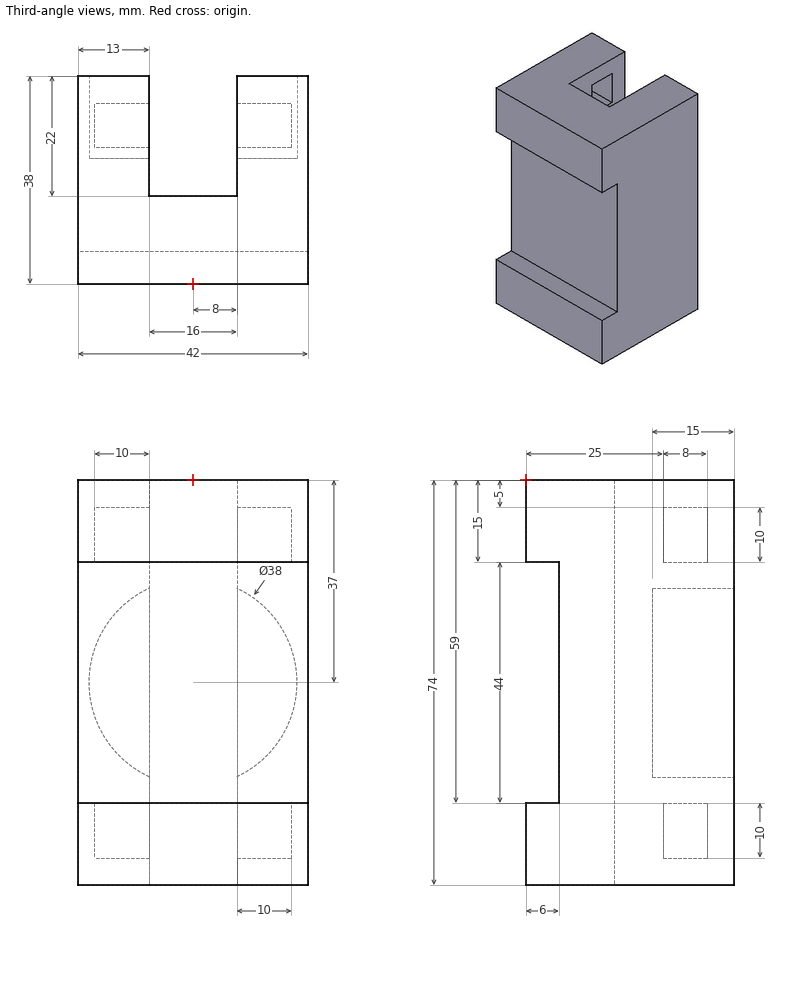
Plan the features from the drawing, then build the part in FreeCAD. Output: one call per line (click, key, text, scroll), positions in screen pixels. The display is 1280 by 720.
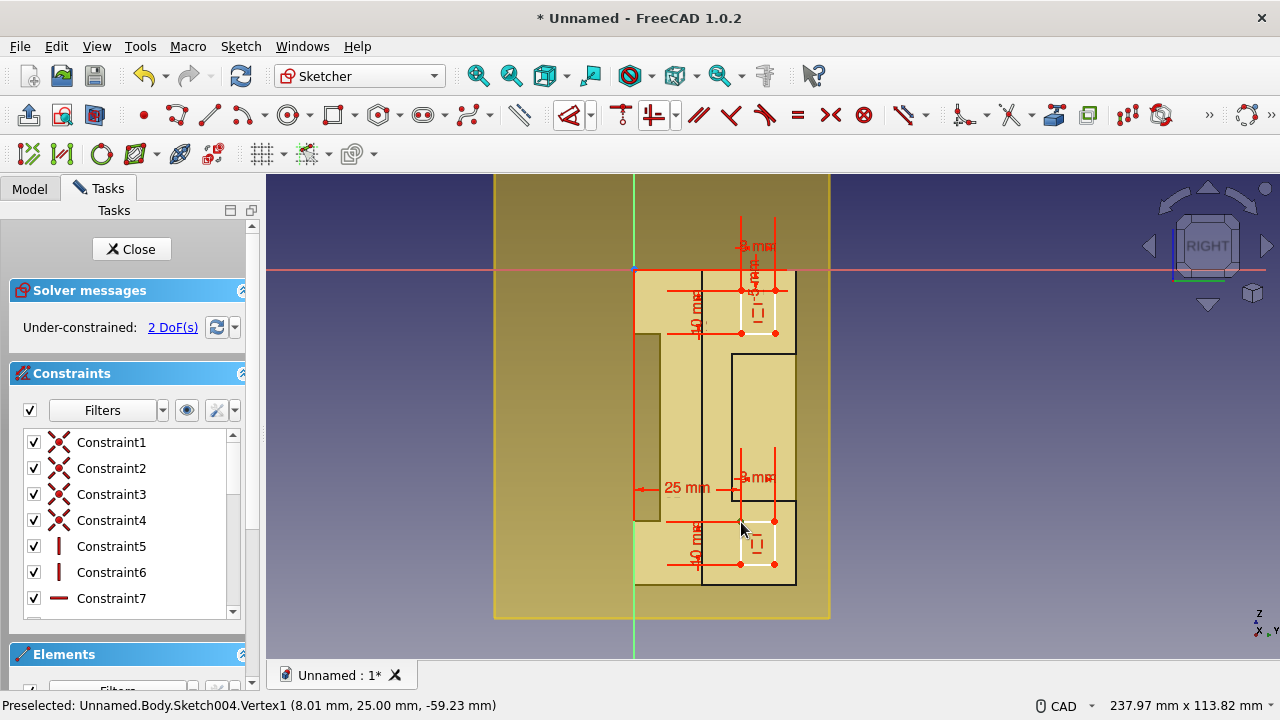
key(i)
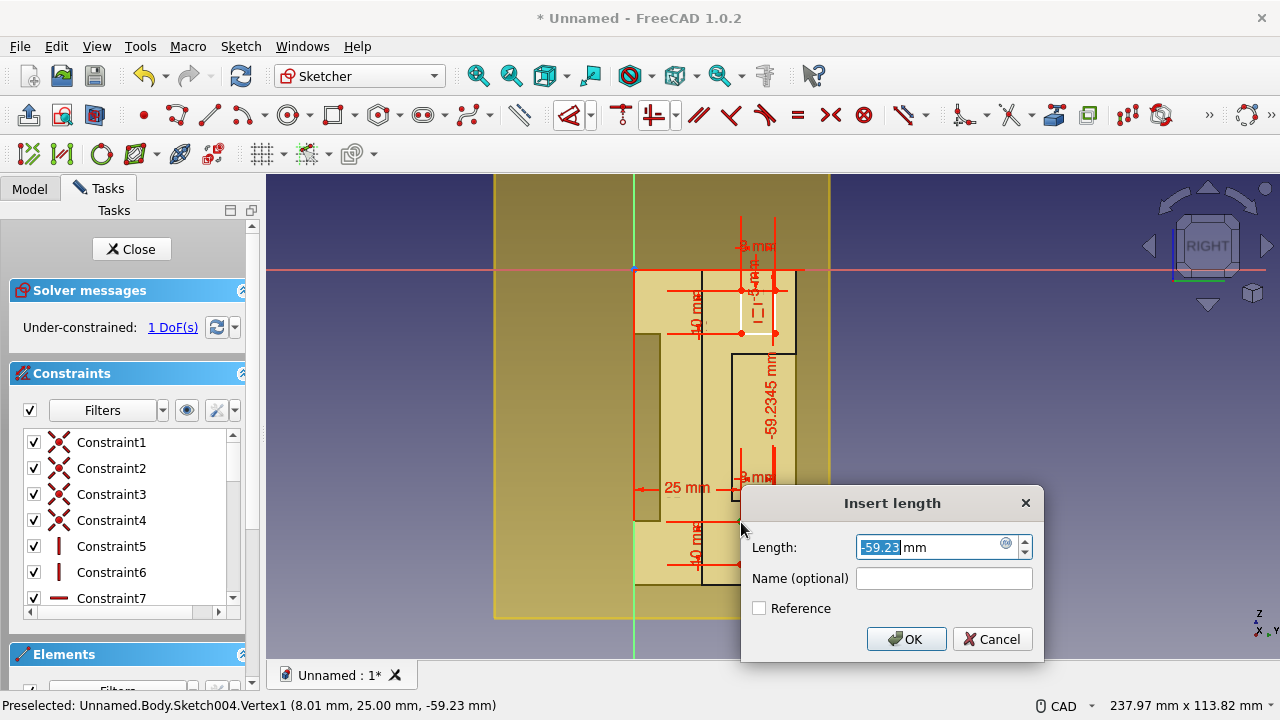
text(-59)
key(Return)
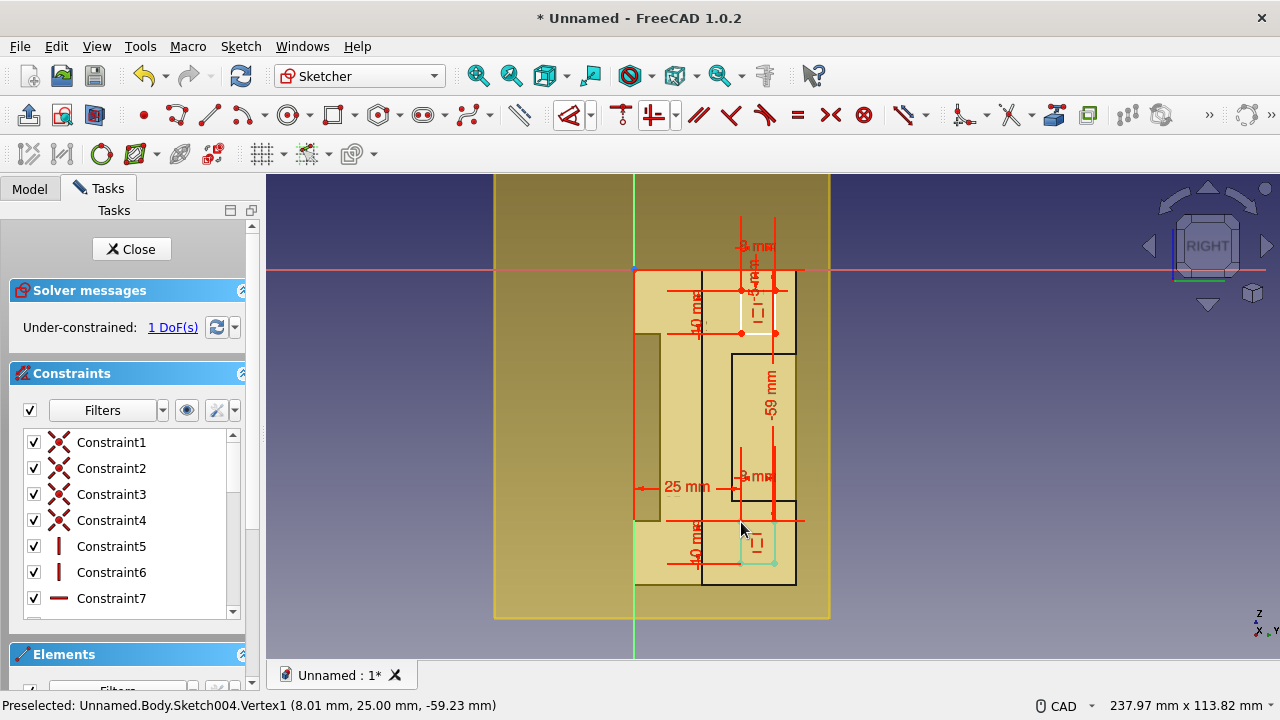
click(741, 291)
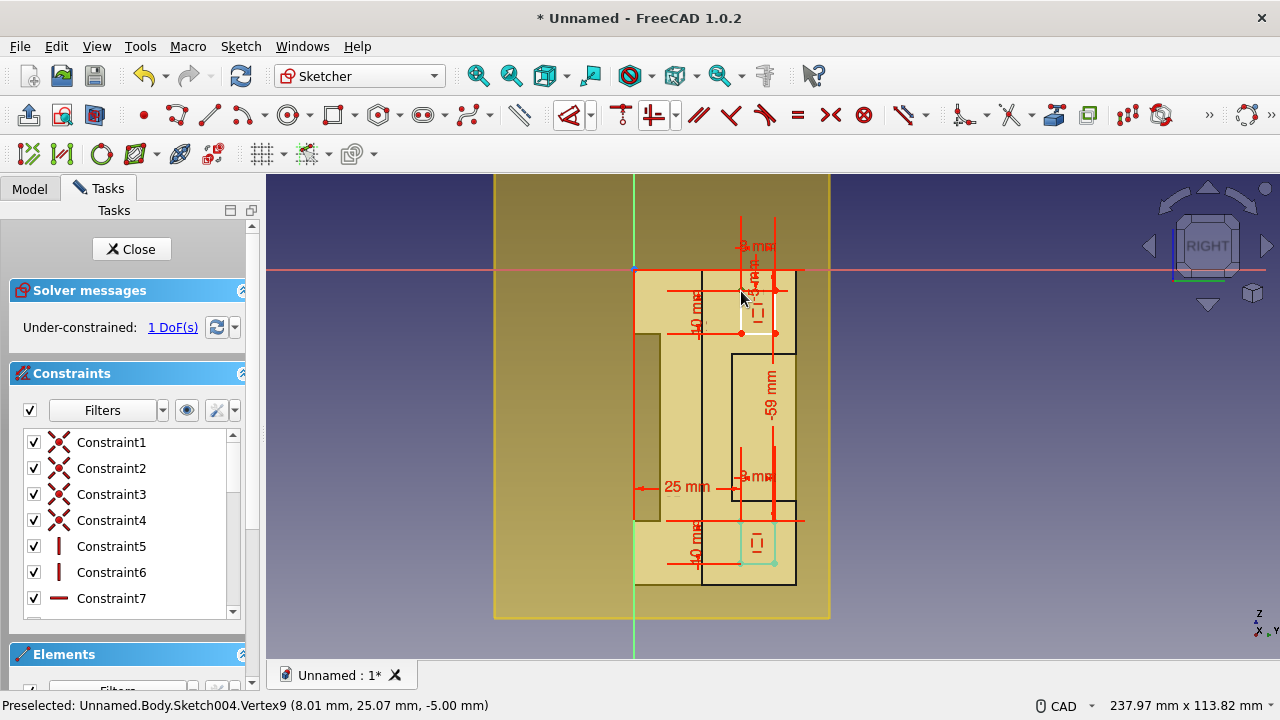
click(590, 116)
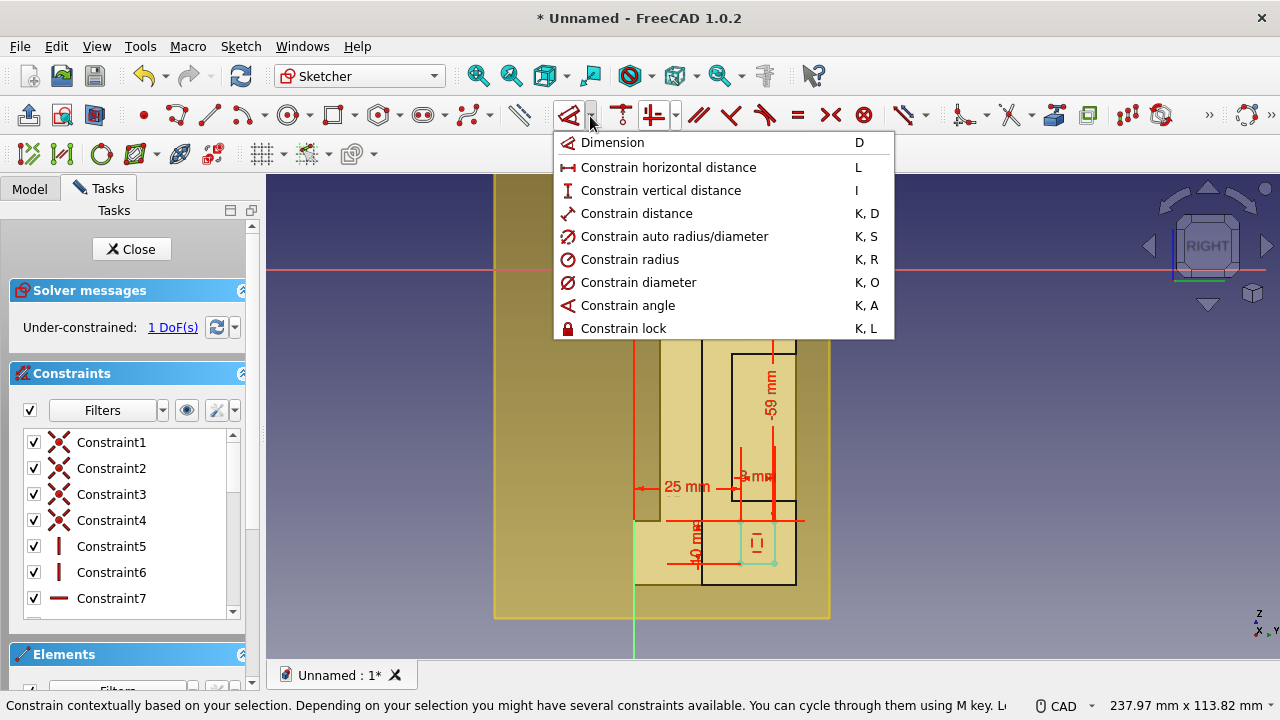
click(724, 168)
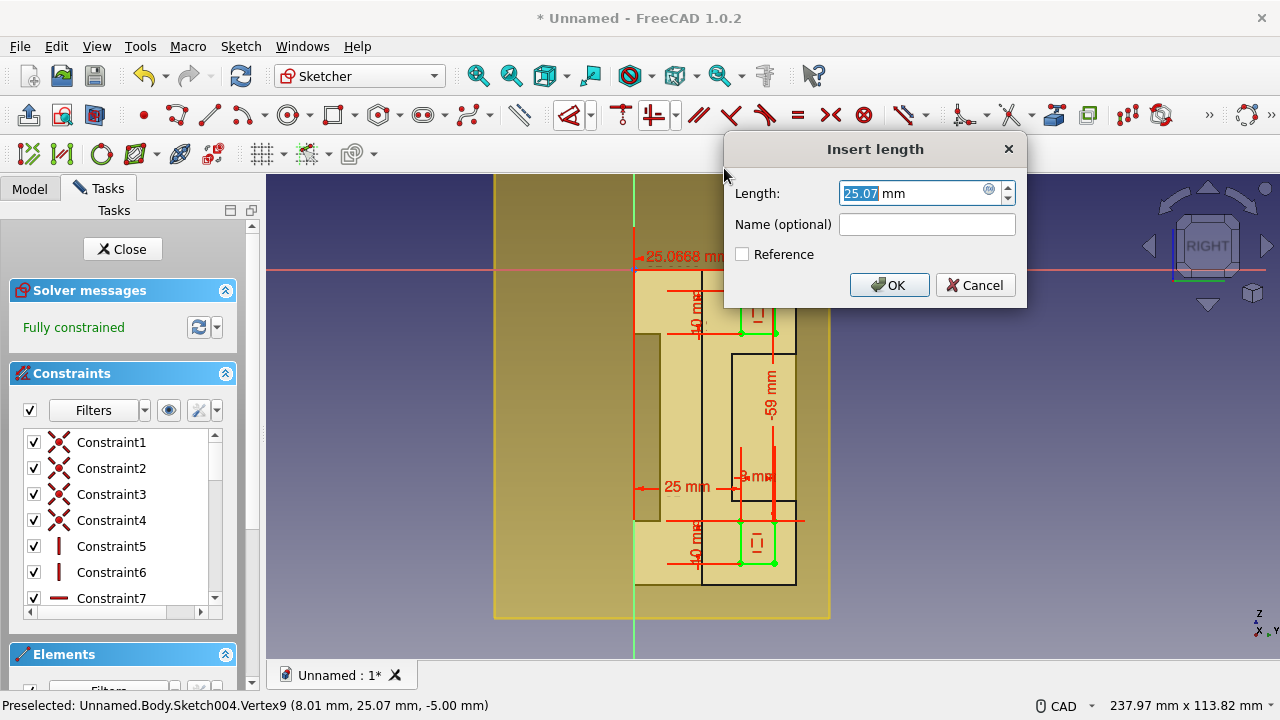
text(25)
key(Return)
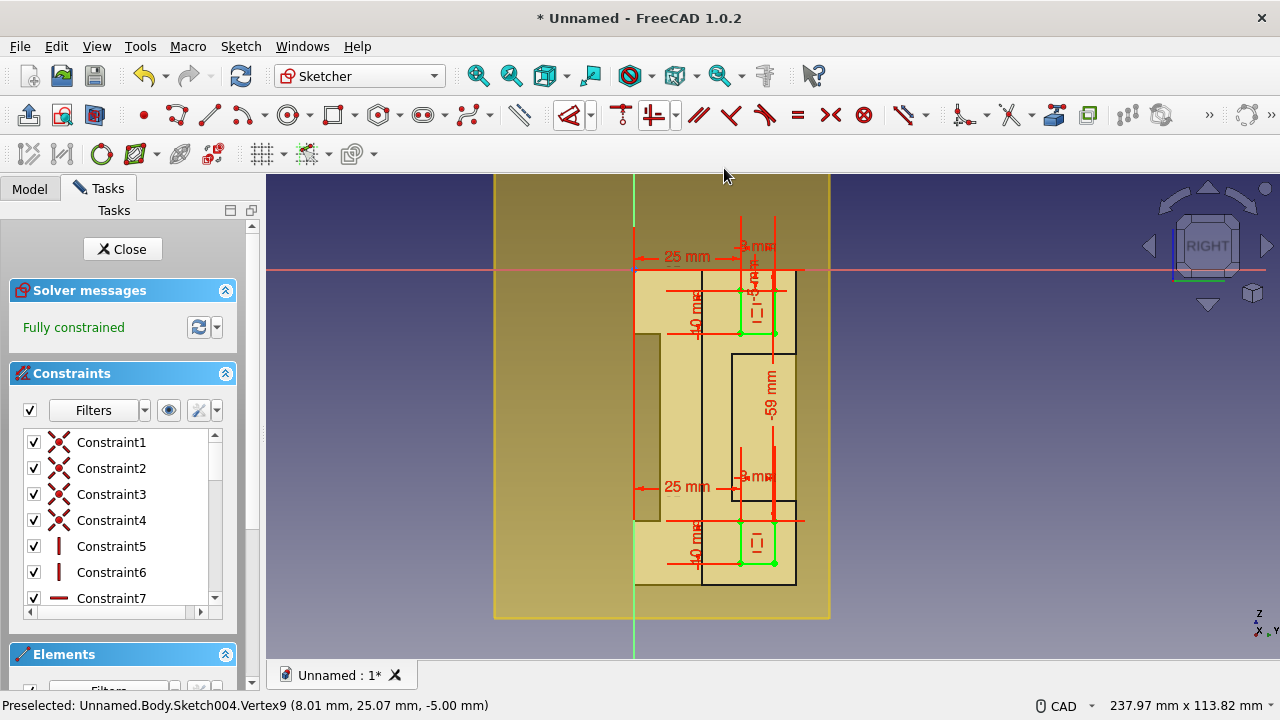
click(123, 249)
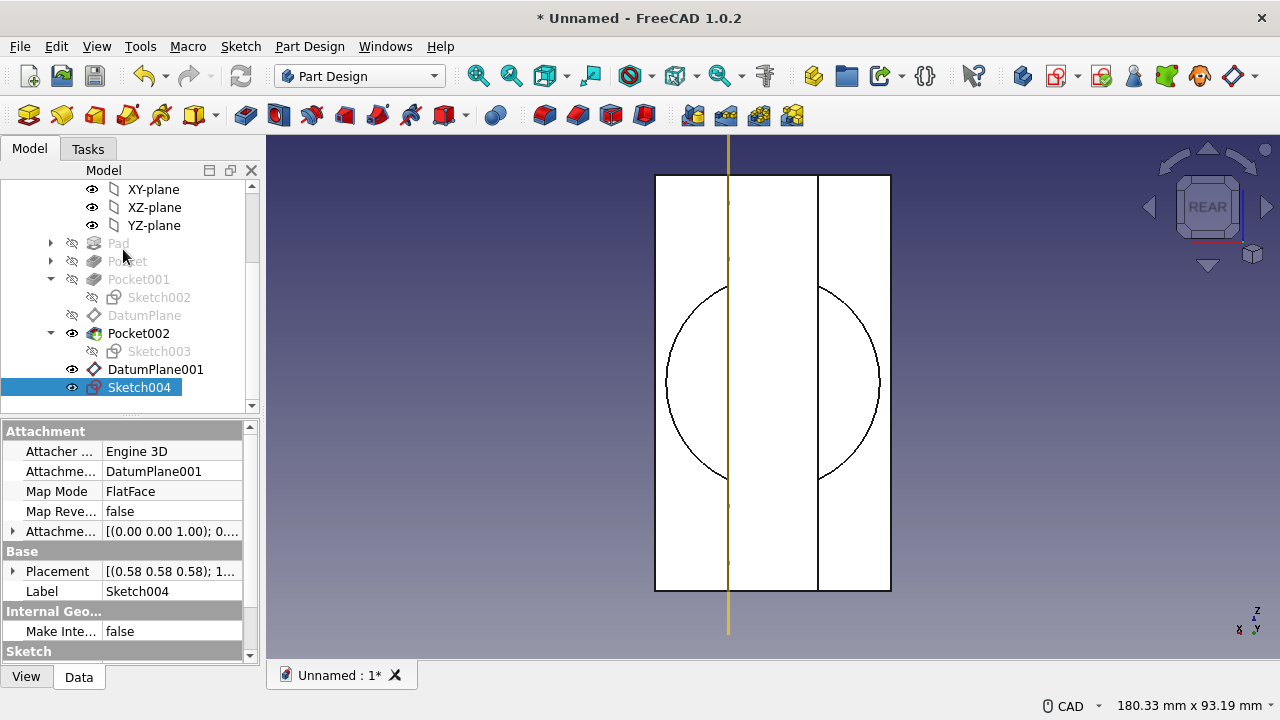
click(246, 116)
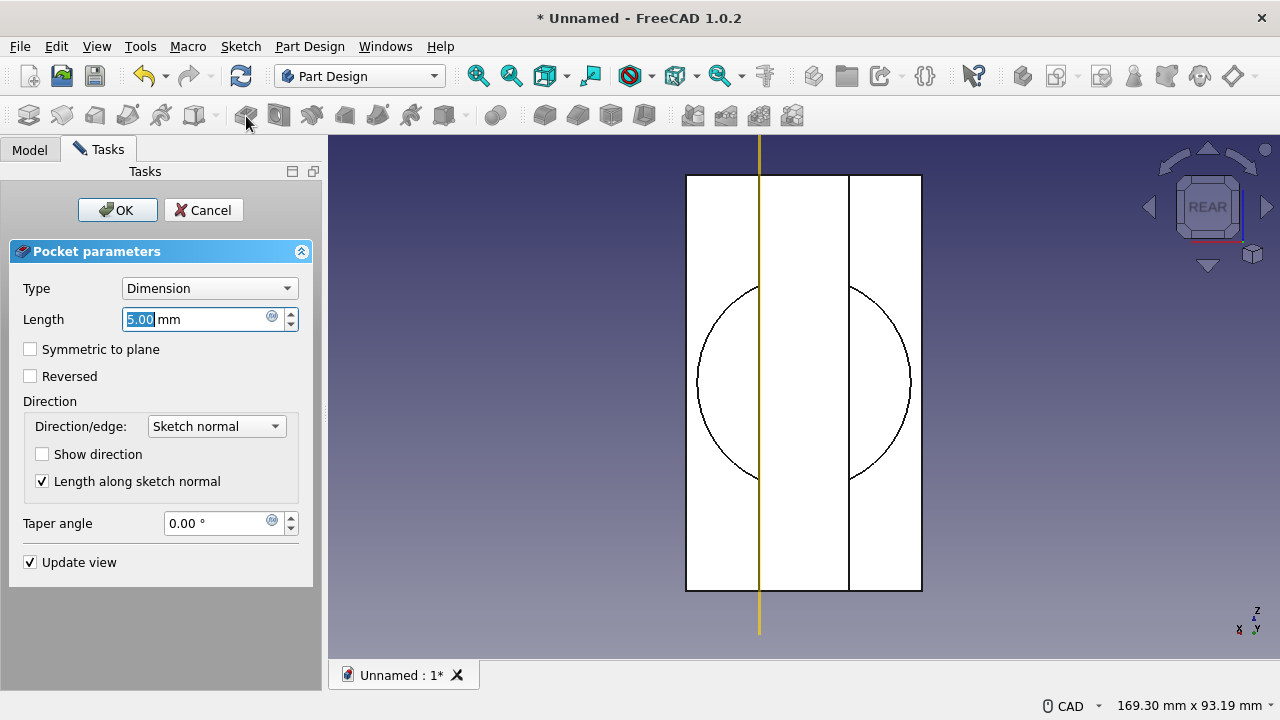
text(10)
key(Tab)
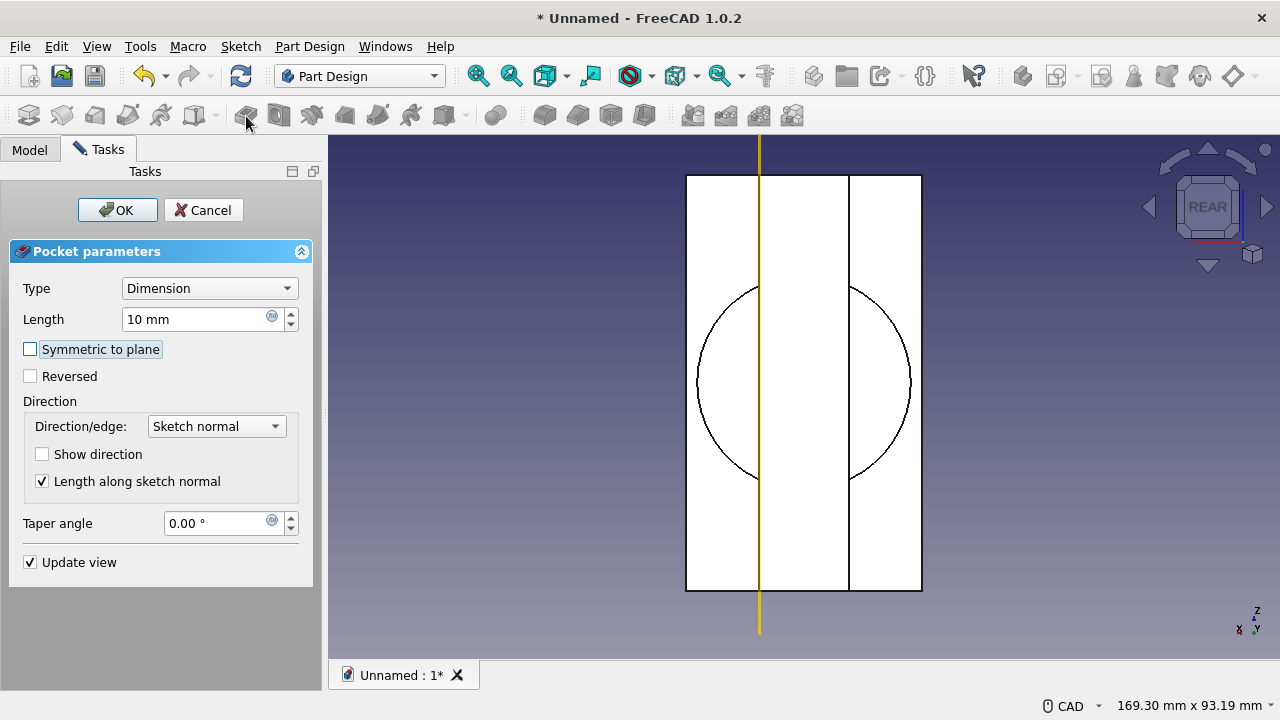
click(31, 376)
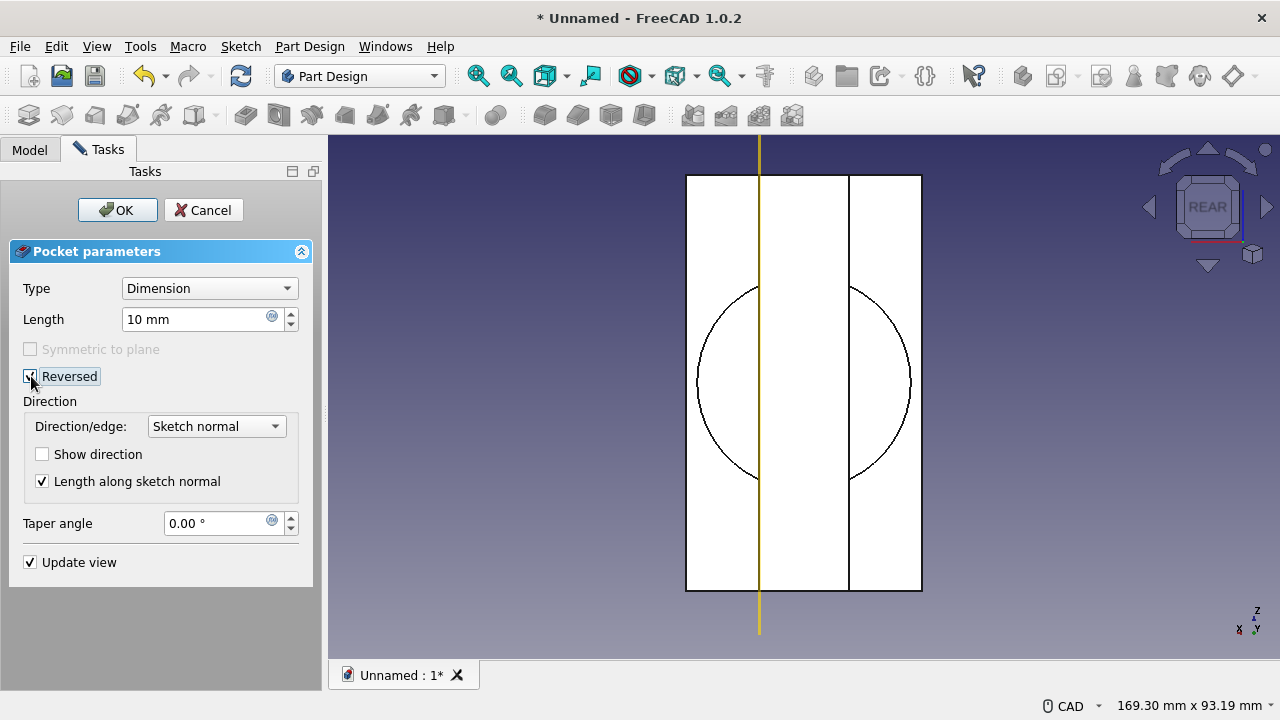
click(118, 210)